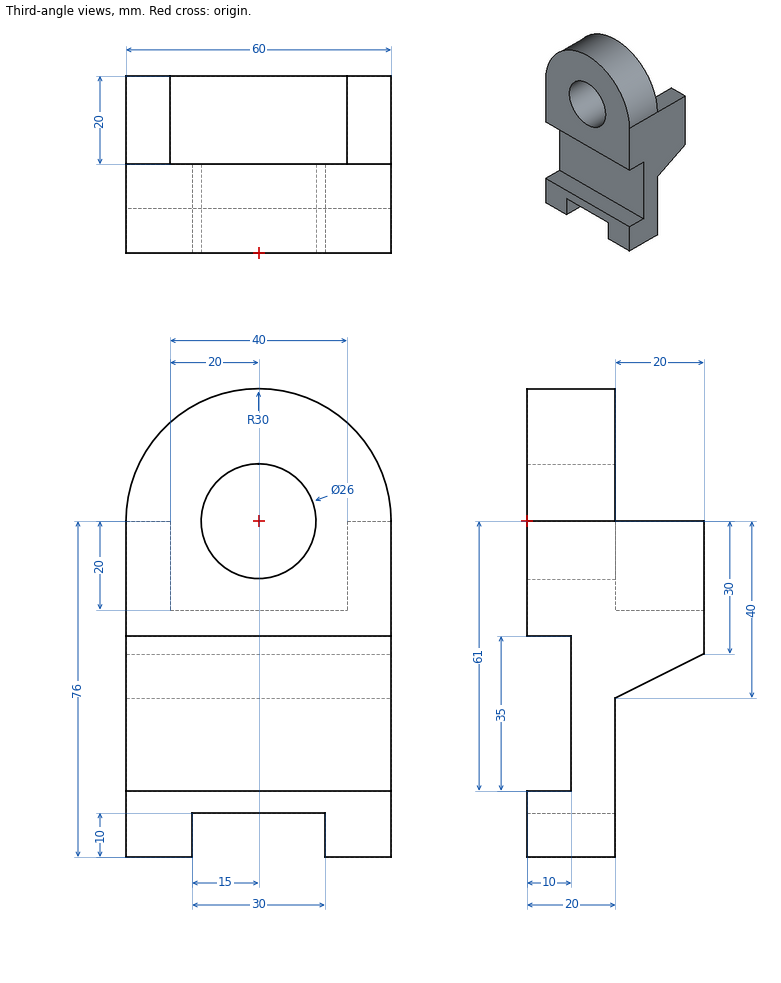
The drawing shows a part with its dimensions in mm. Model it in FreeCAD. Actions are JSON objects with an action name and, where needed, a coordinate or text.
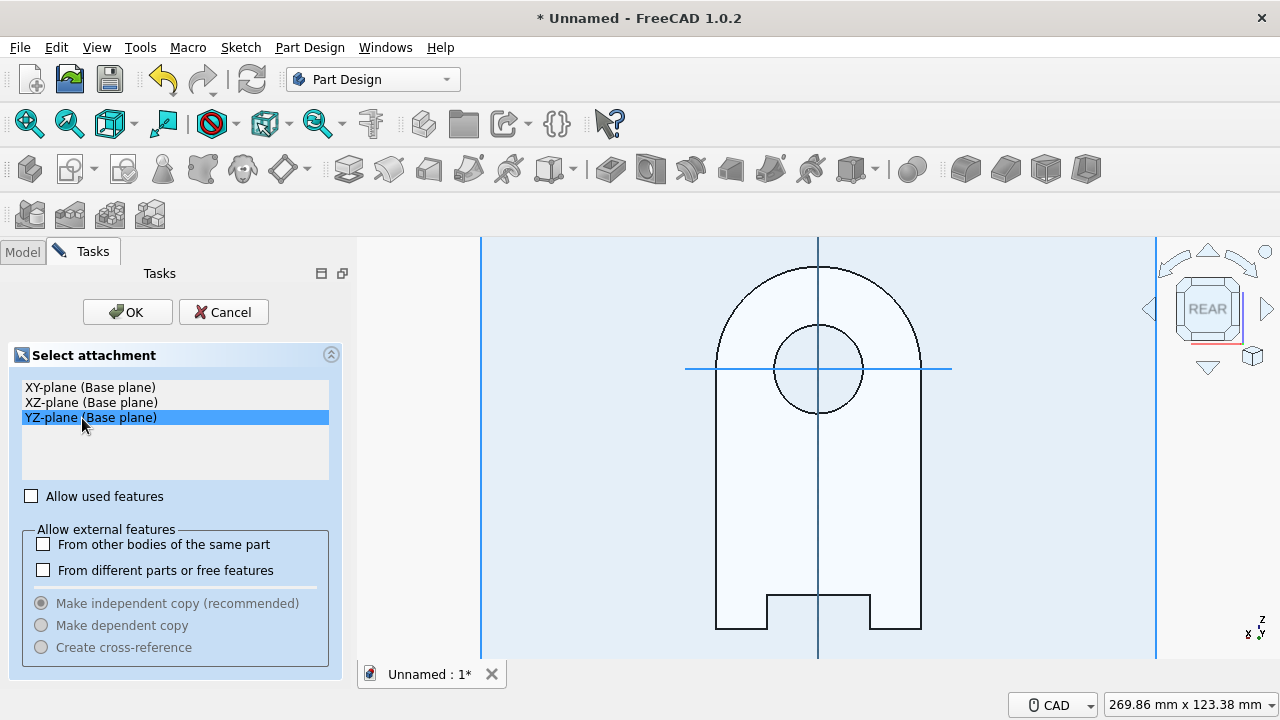
{"action": "left_click", "coordinate": [128, 312]}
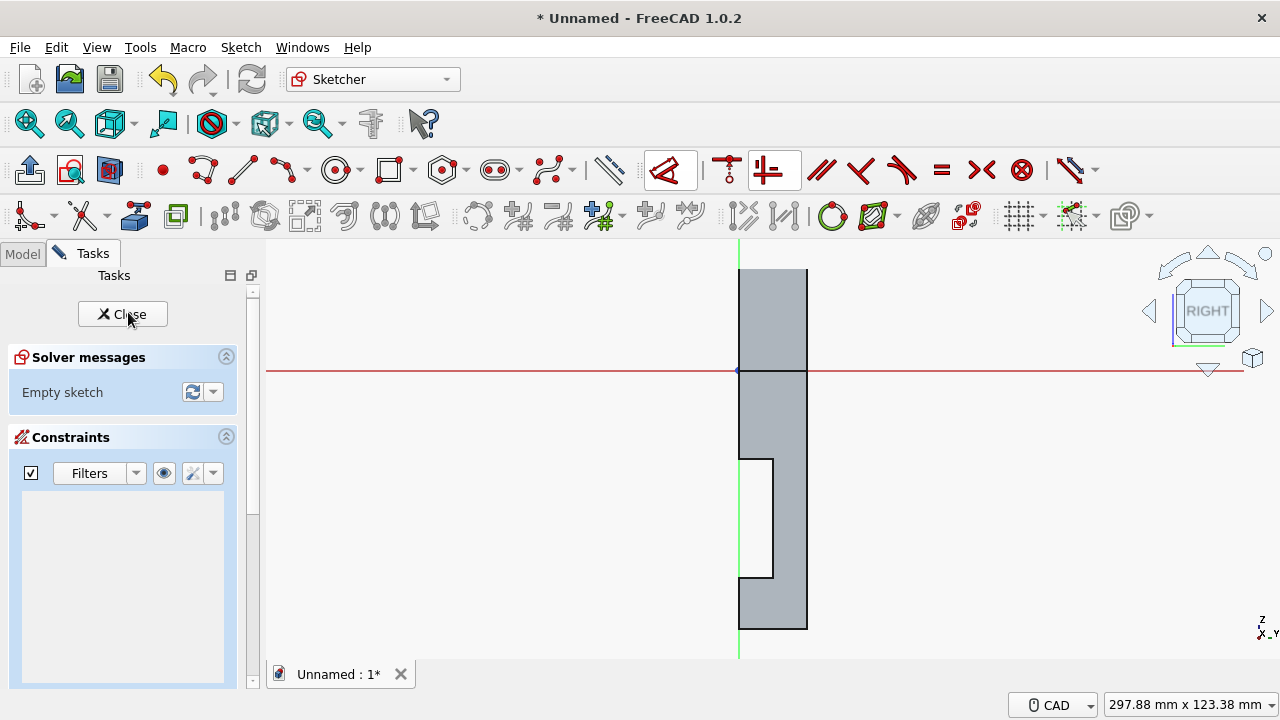
{"action": "key", "text": "q s"}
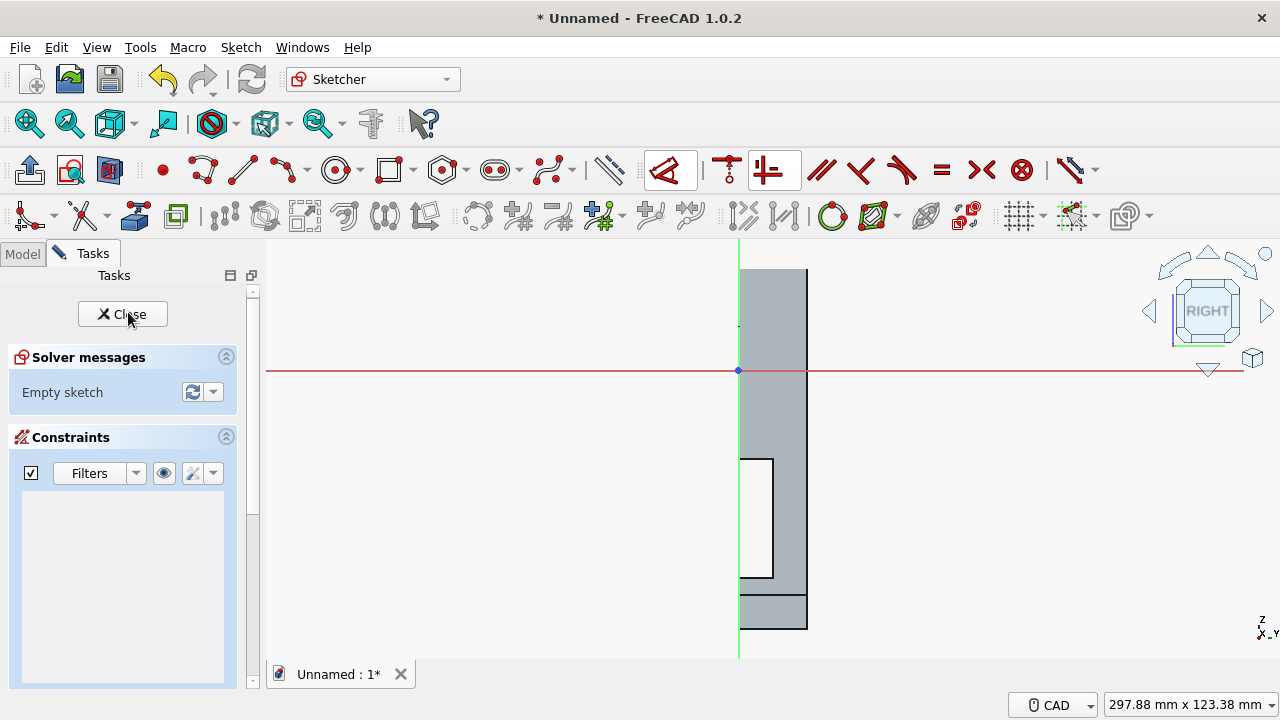
{"action": "scroll", "coordinate": [932, 426], "scroll_direction": "up", "scroll_amount": 3}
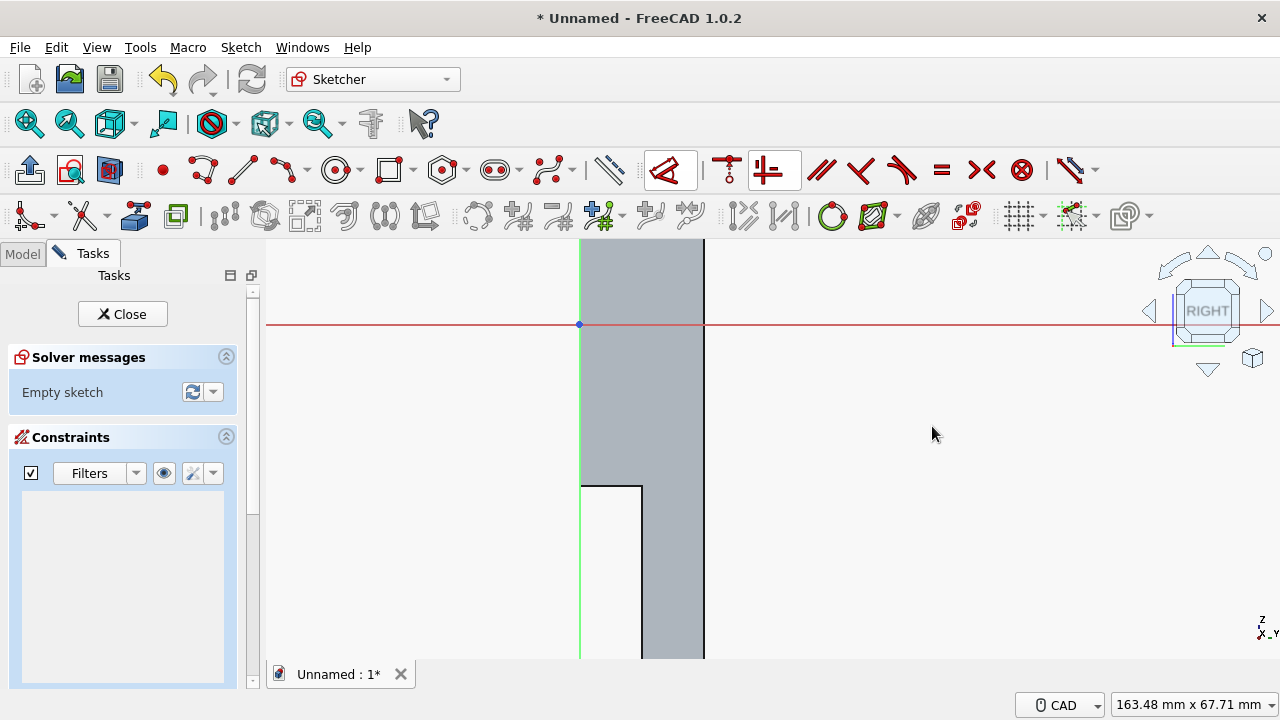
{"action": "left_click", "coordinate": [204, 170]}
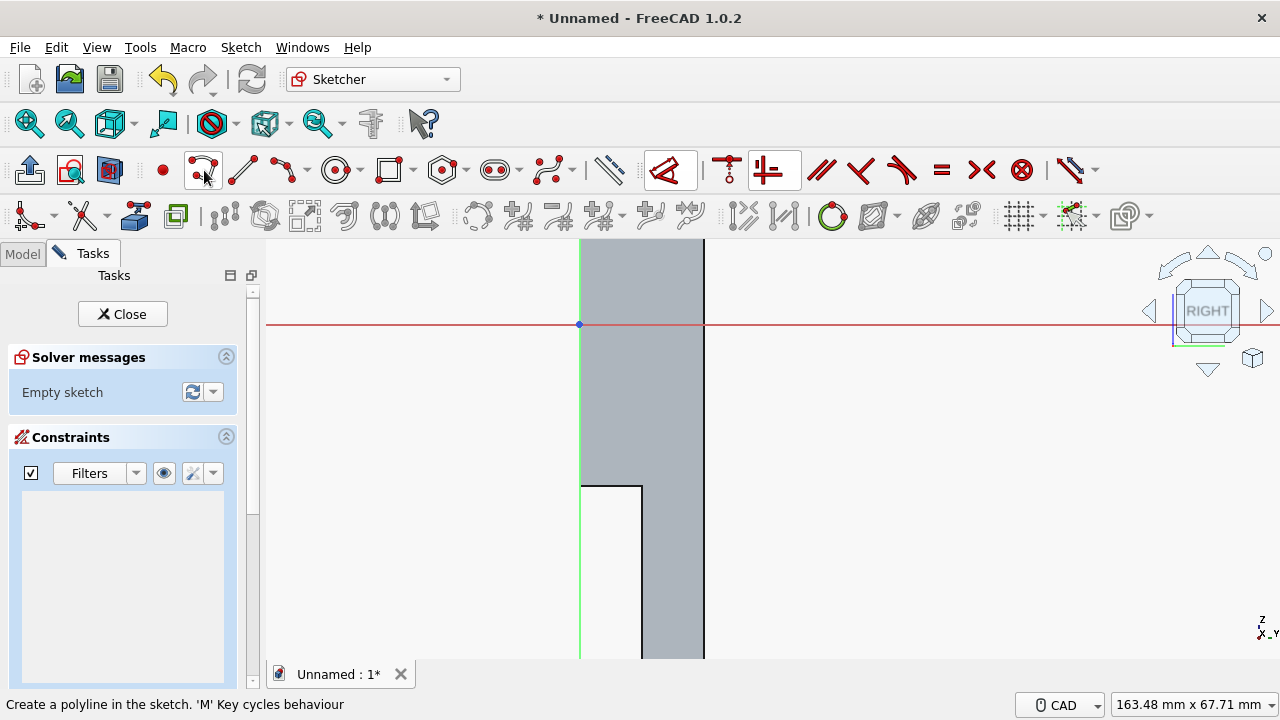
{"action": "left_click", "coordinate": [704, 325]}
{"action": "left_click", "coordinate": [704, 573]}
{"action": "left_click", "coordinate": [828, 511]}
{"action": "left_click", "coordinate": [828, 334]}
{"action": "left_click", "coordinate": [704, 325]}
{"action": "key", "text": "Escape"}
{"action": "key", "text": "Escape"}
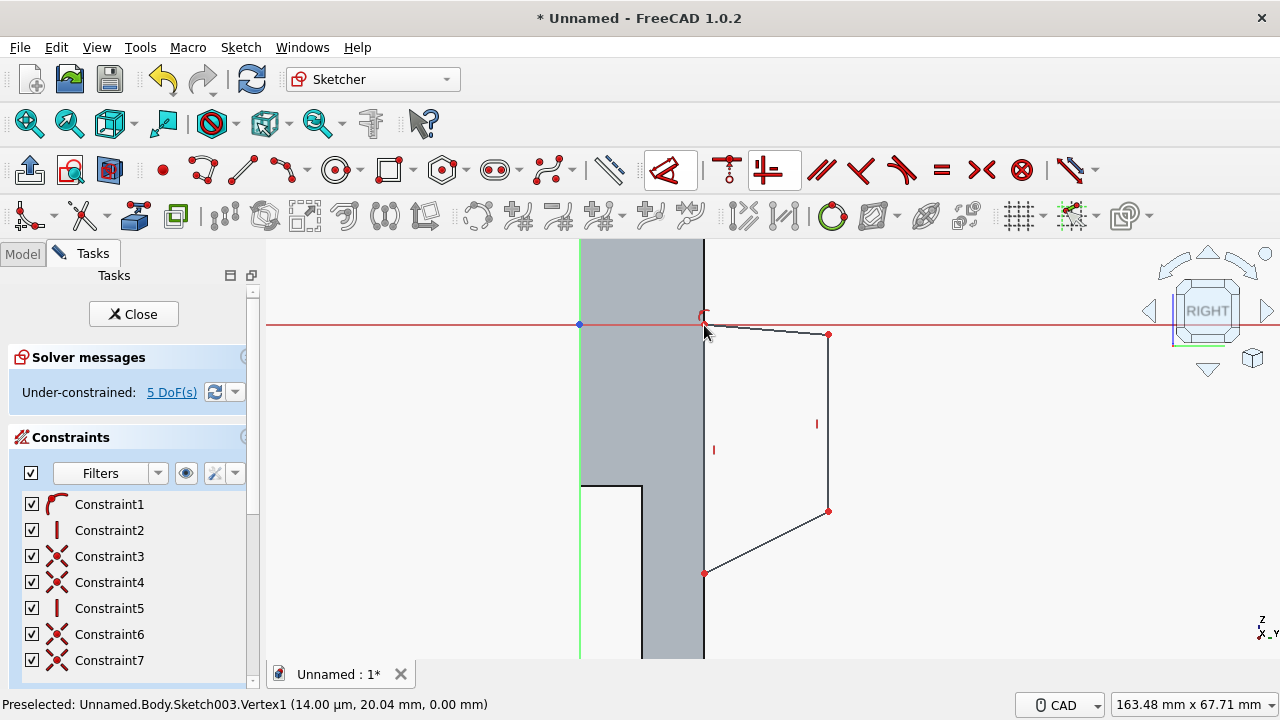
{"action": "left_click", "coordinate": [741, 328]}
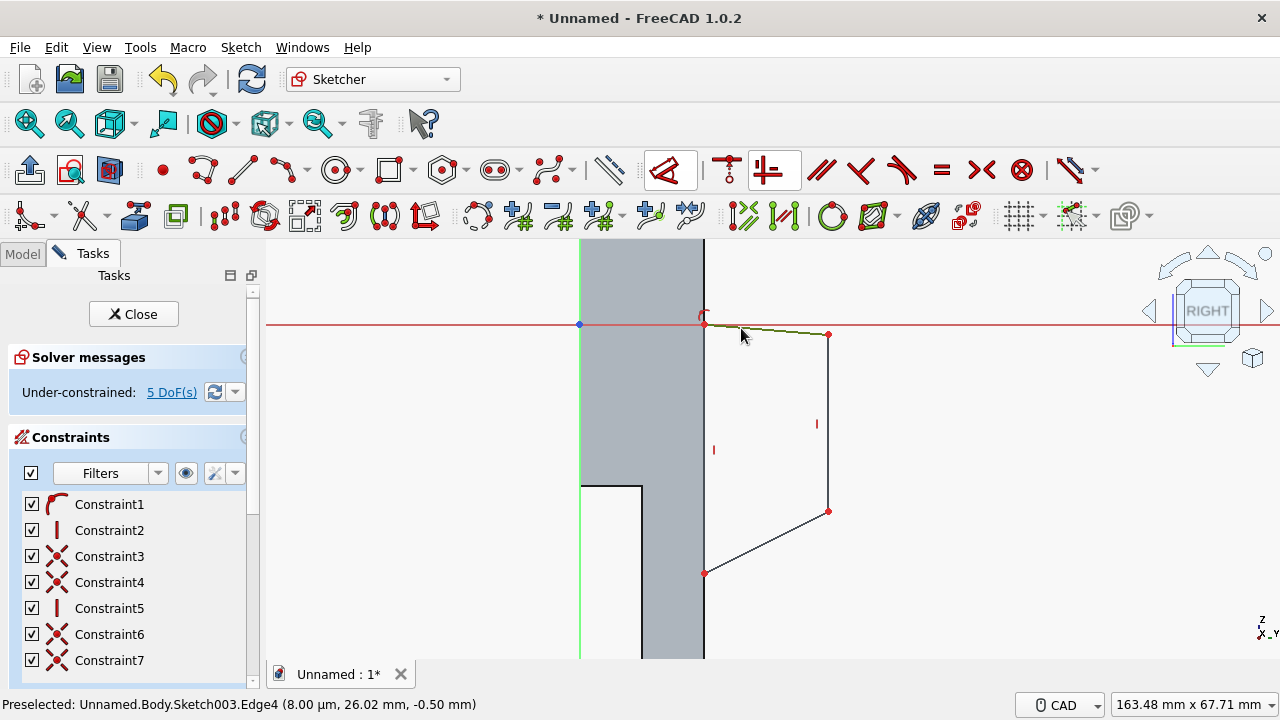
{"action": "key", "text": "h"}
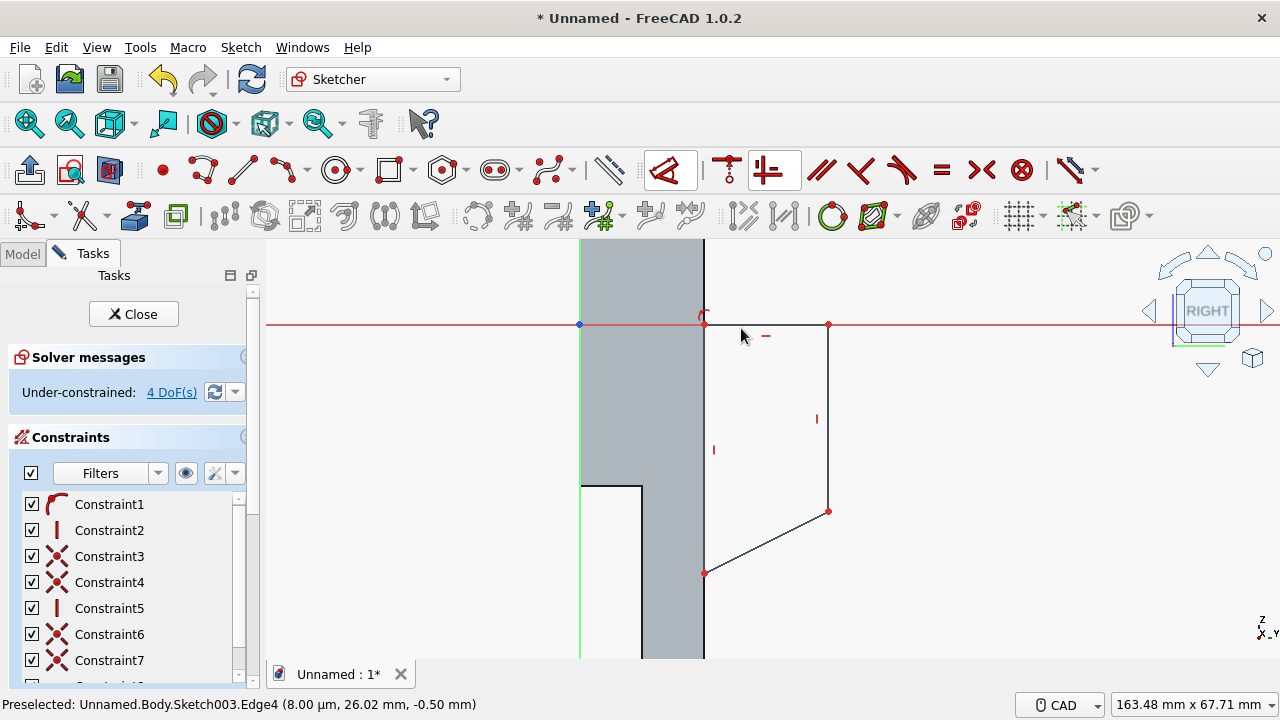
{"action": "left_click", "coordinate": [704, 399]}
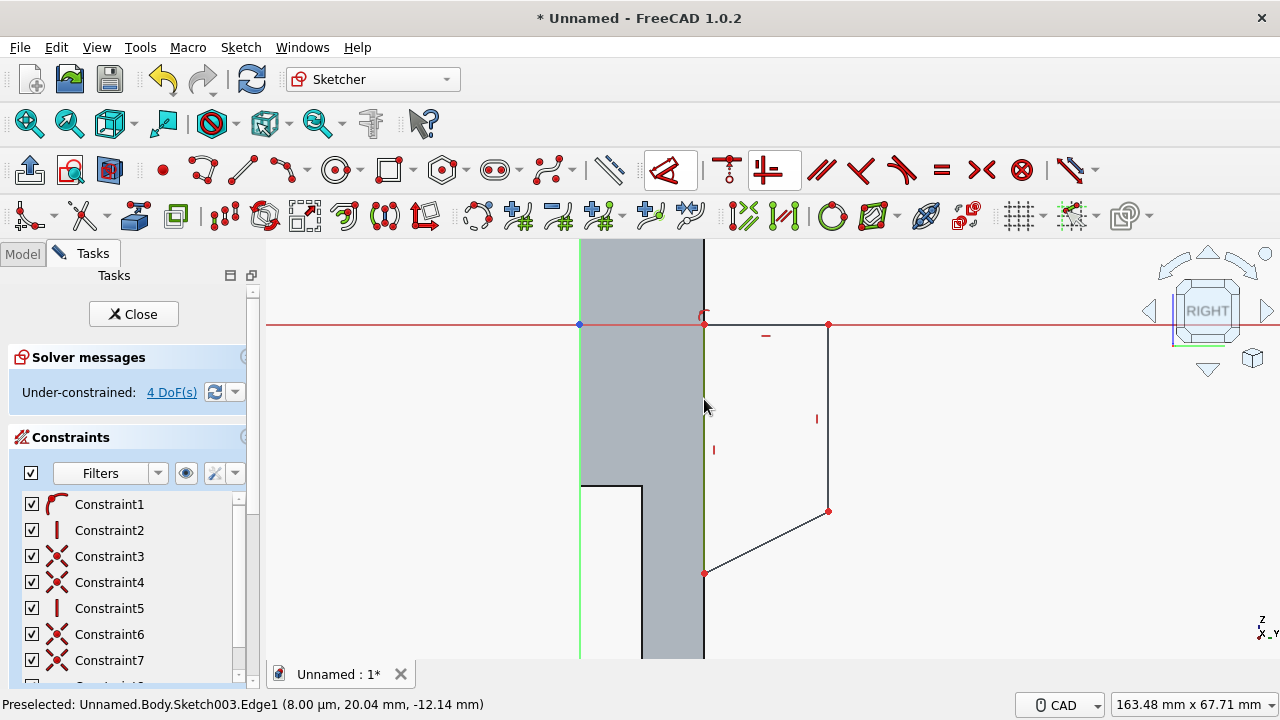
{"action": "left_click", "coordinate": [692, 170]}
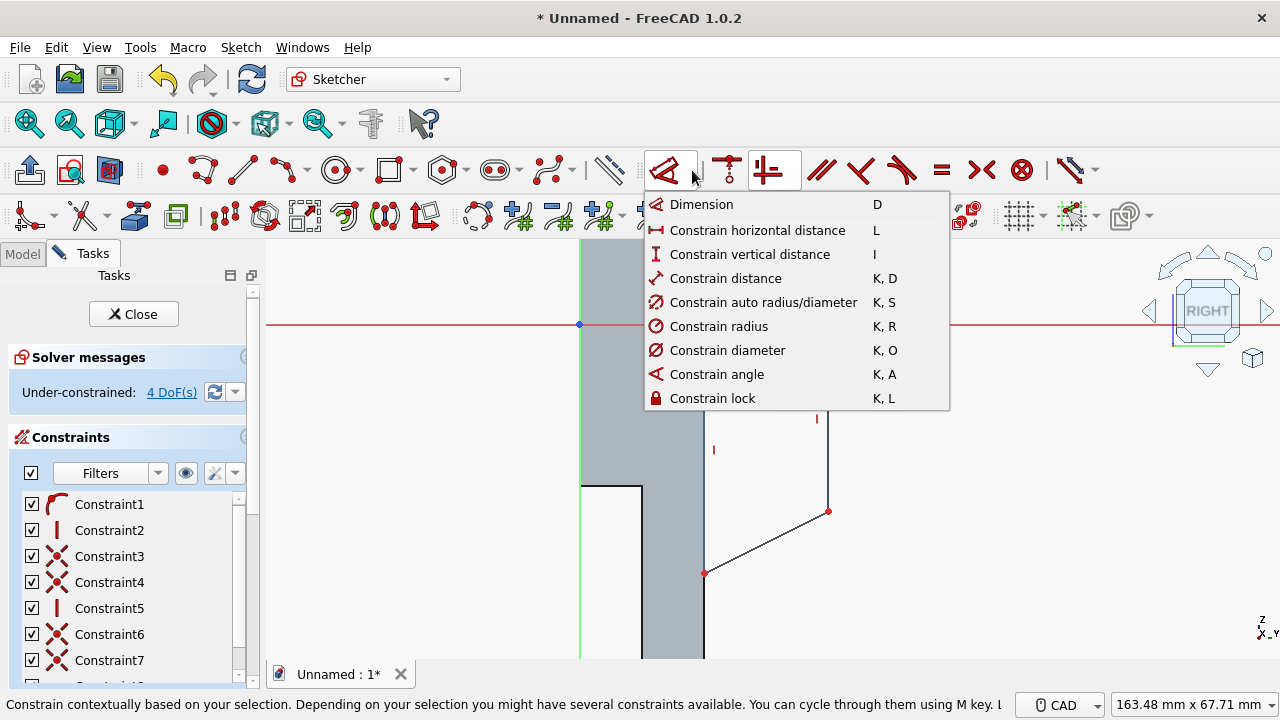
{"action": "left_click", "coordinate": [797, 254]}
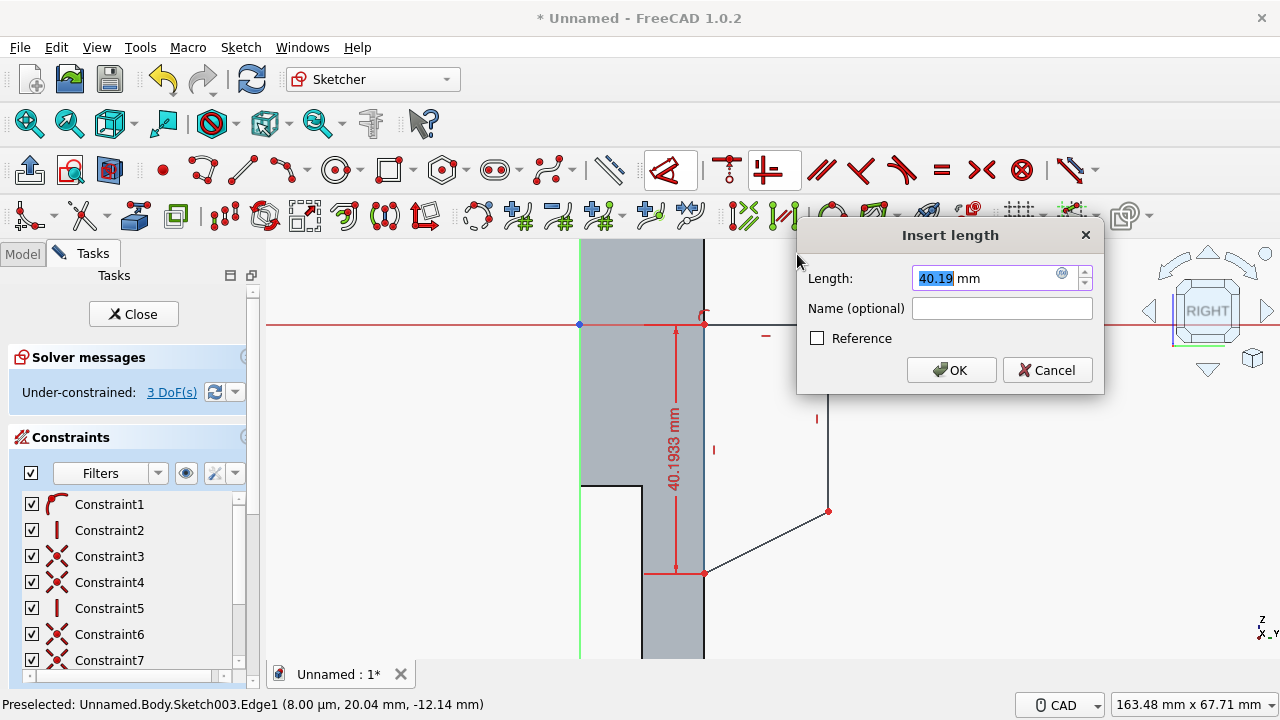
{"action": "type", "text": "40"}
{"action": "key", "text": "Return"}